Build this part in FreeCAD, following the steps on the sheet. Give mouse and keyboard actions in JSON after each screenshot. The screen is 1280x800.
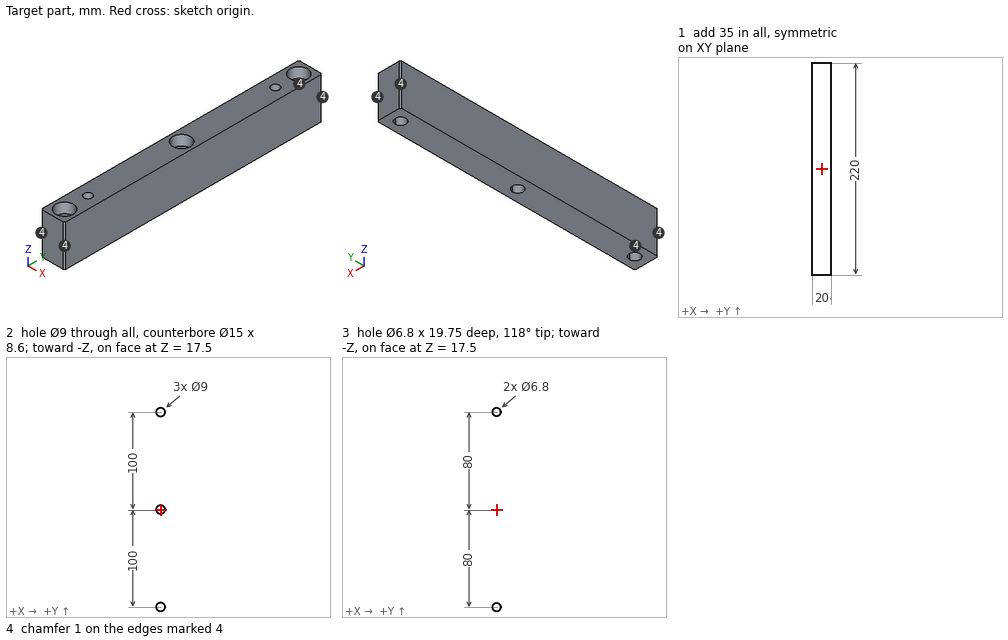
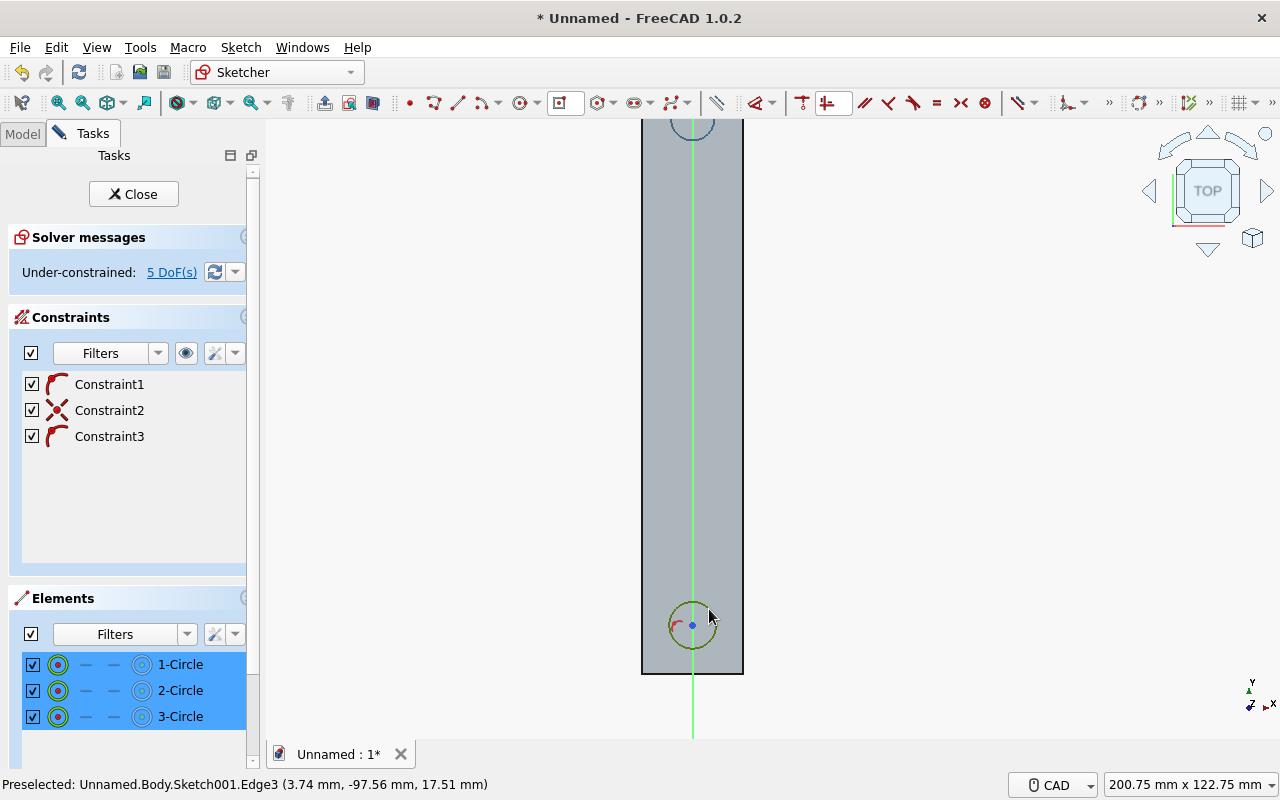
{"action": "key", "text": "e"}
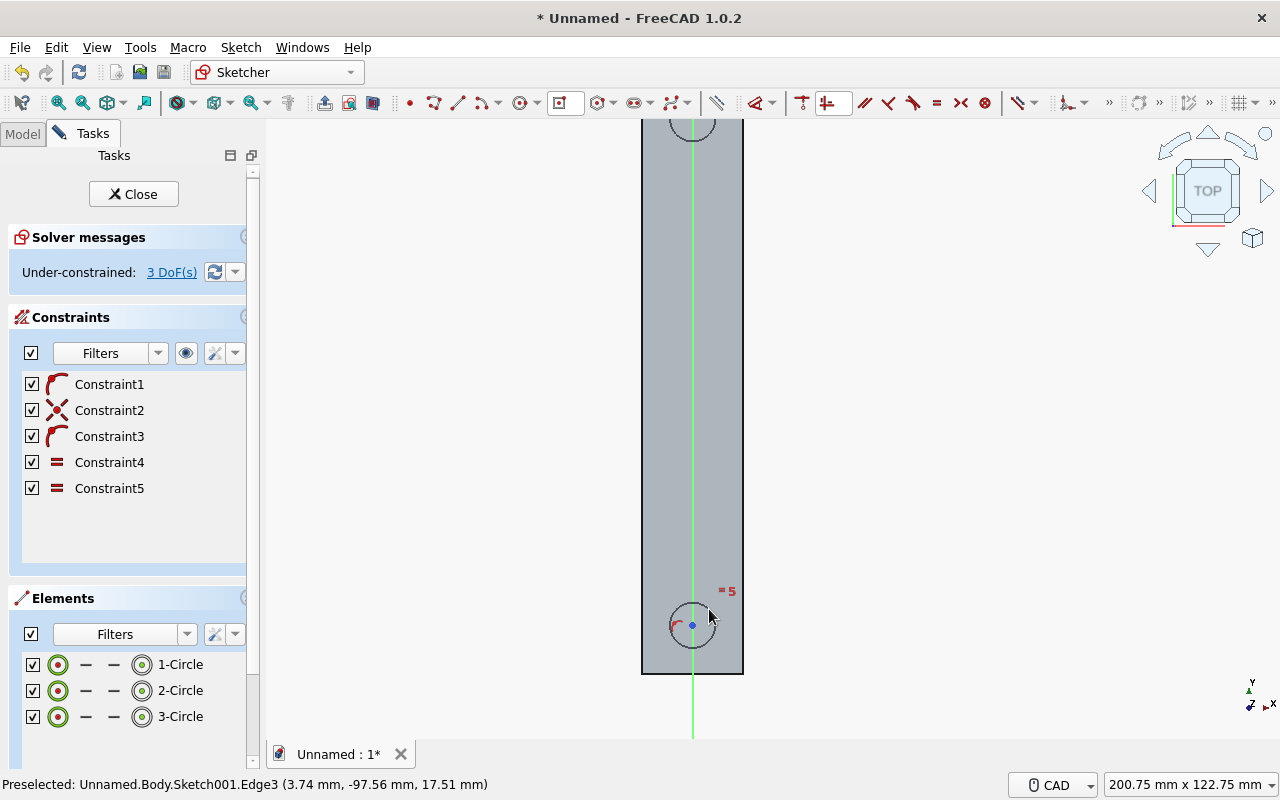
{"action": "left_click", "coordinate": [756, 104]}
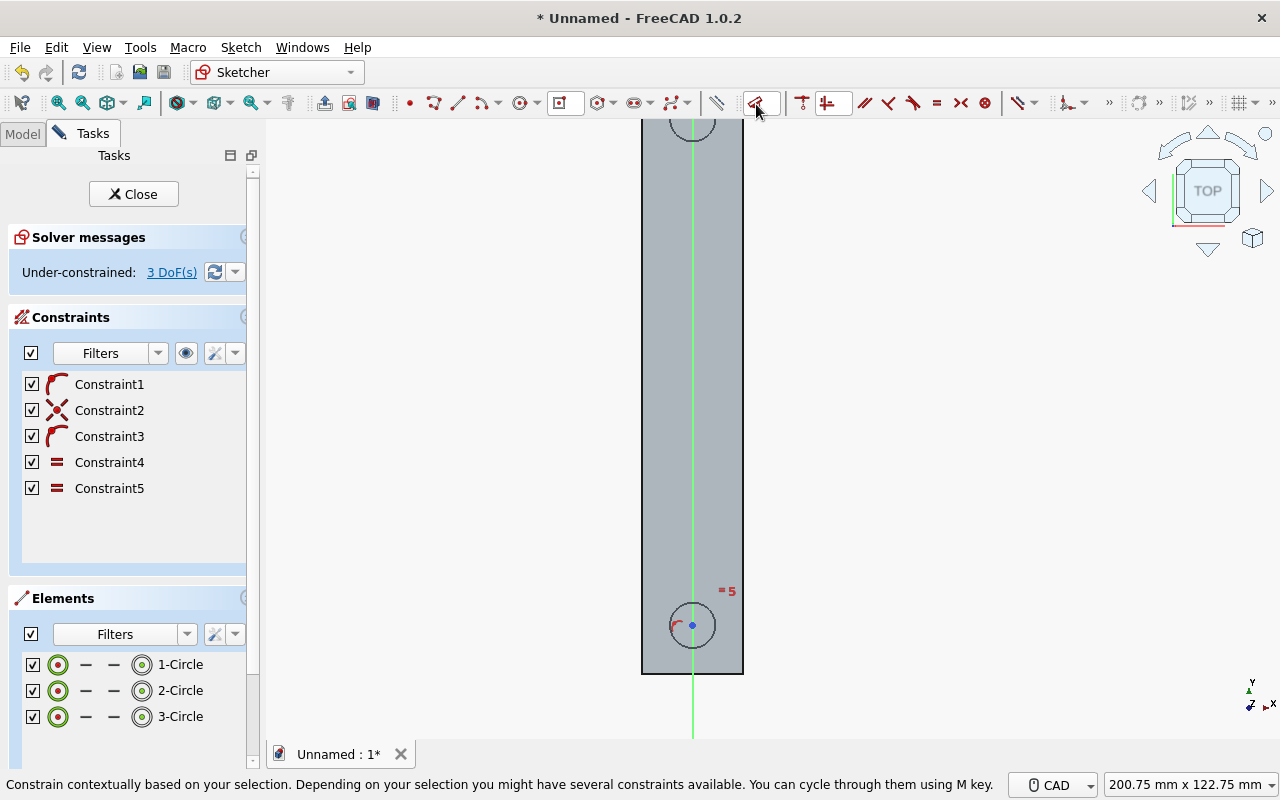
{"action": "scroll", "coordinate": [711, 610], "scroll_direction": "down", "scroll_amount": 5}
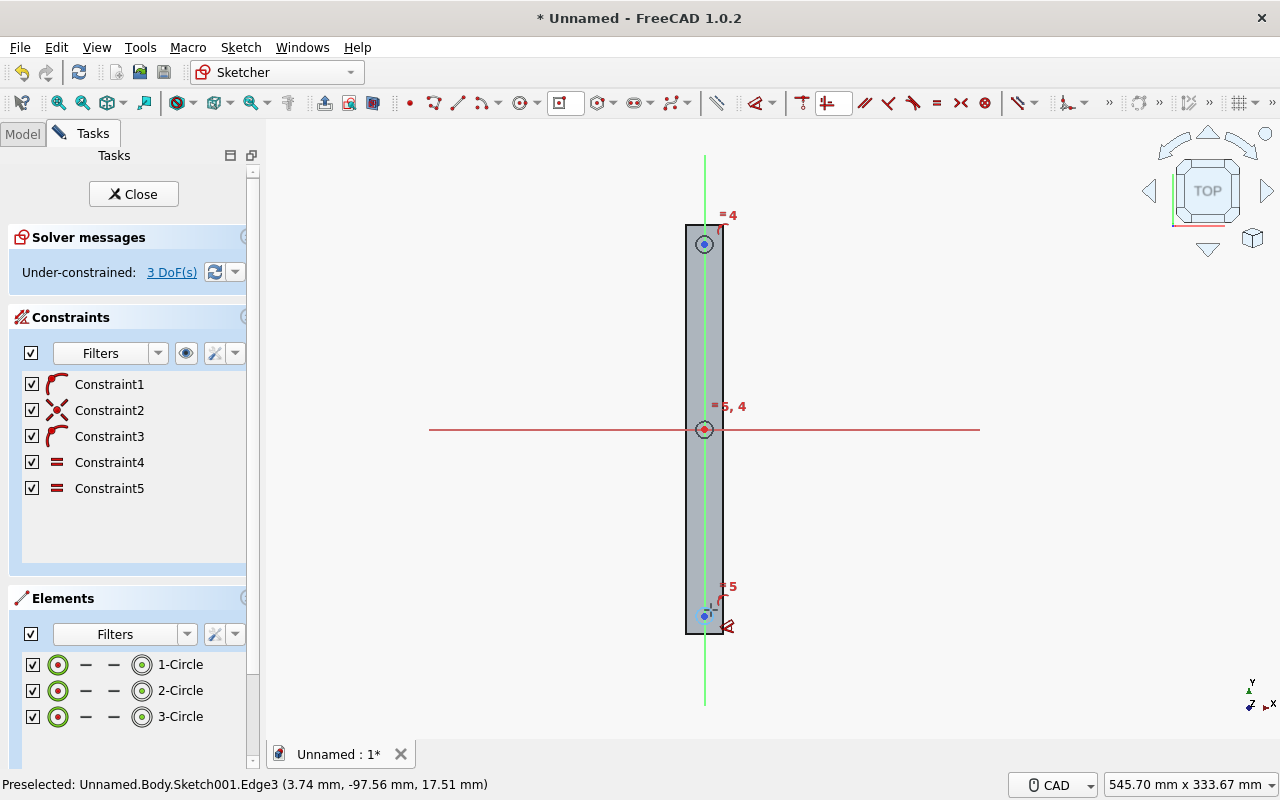
{"action": "scroll", "coordinate": [710, 239], "scroll_direction": "up", "scroll_amount": 5}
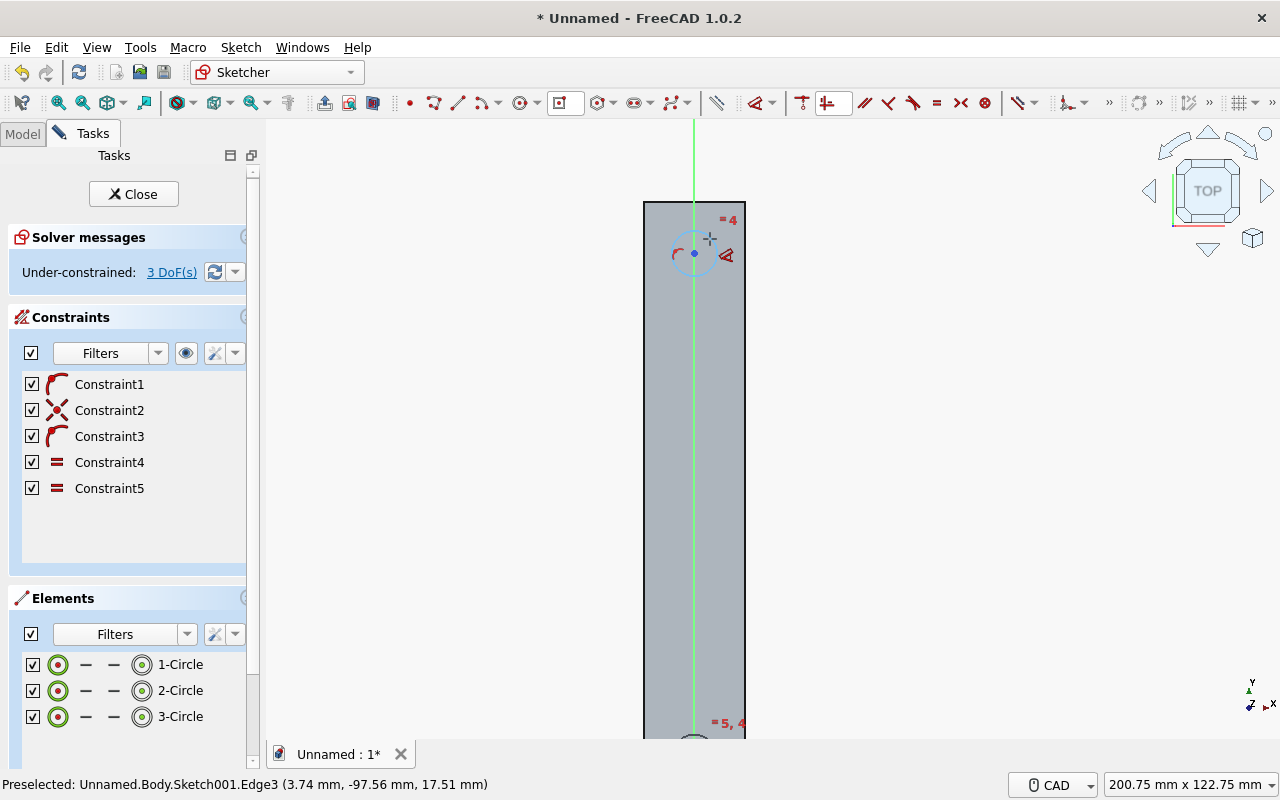
{"action": "left_click", "coordinate": [710, 238]}
{"action": "left_click", "coordinate": [733, 215]}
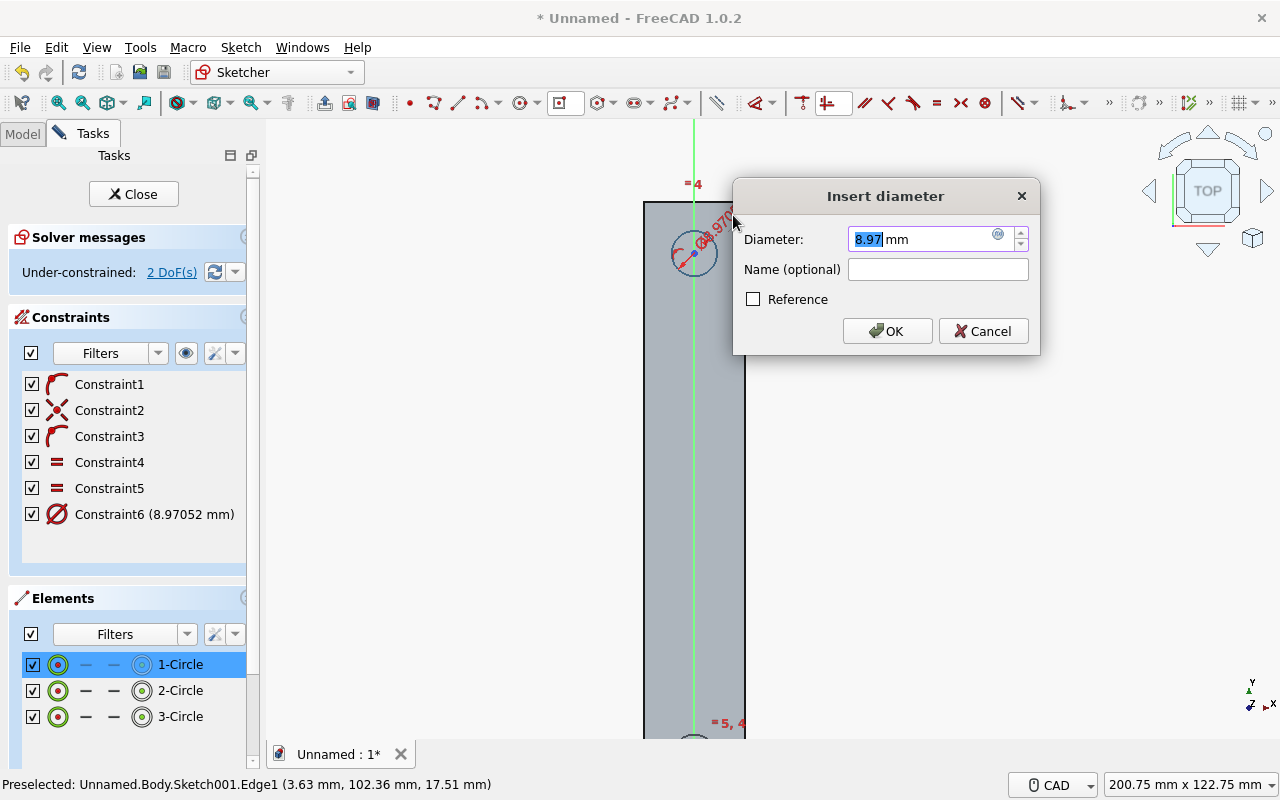
{"action": "type", "text": "9"}
{"action": "key", "text": "Return"}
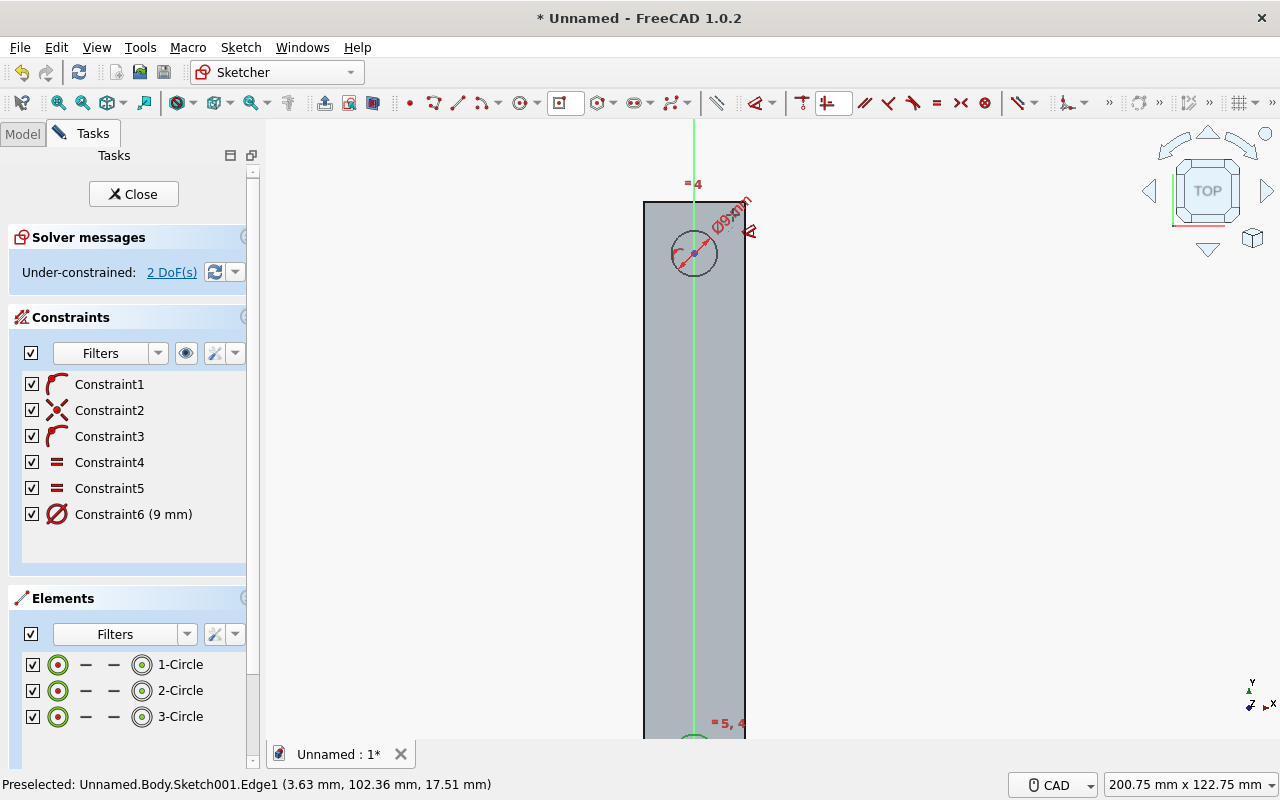
{"action": "left_click", "coordinate": [694, 254]}
{"action": "left_click", "coordinate": [728, 482]}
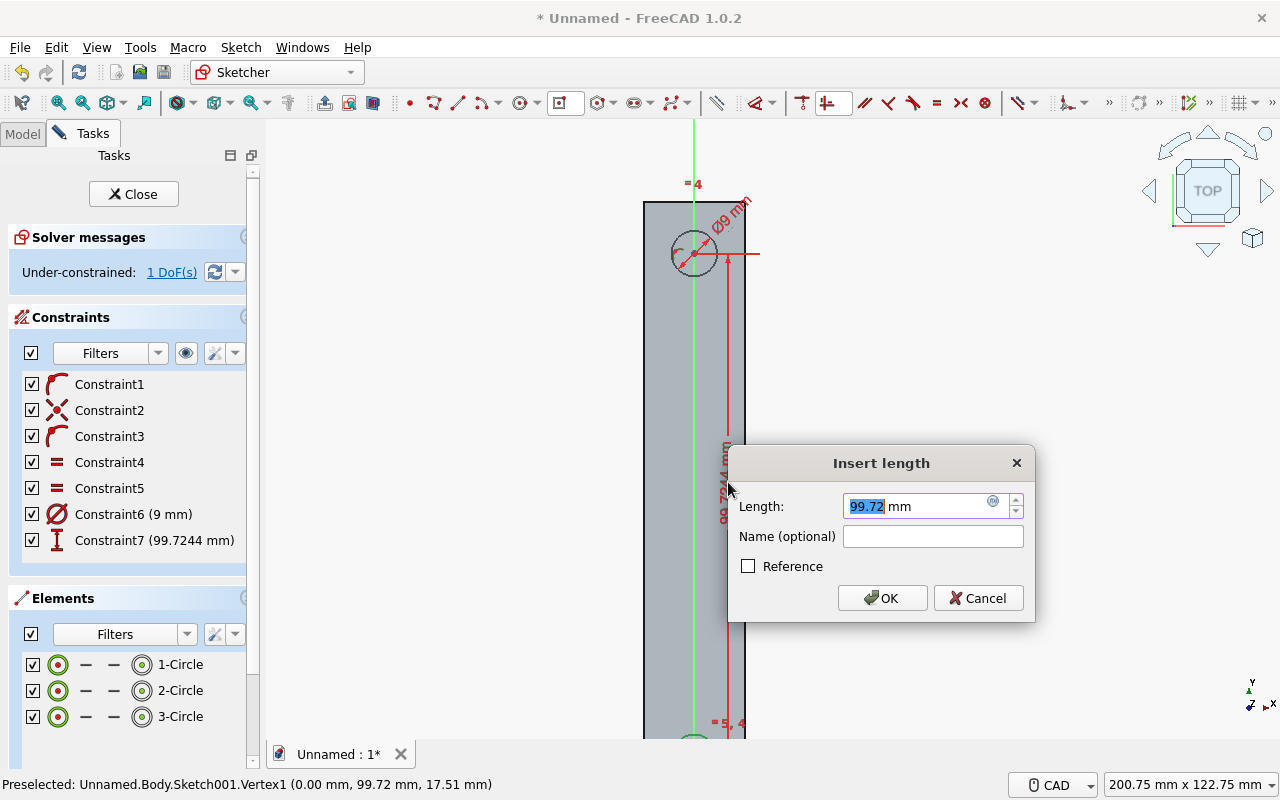
{"action": "type", "text": "100"}
{"action": "key", "text": "Return"}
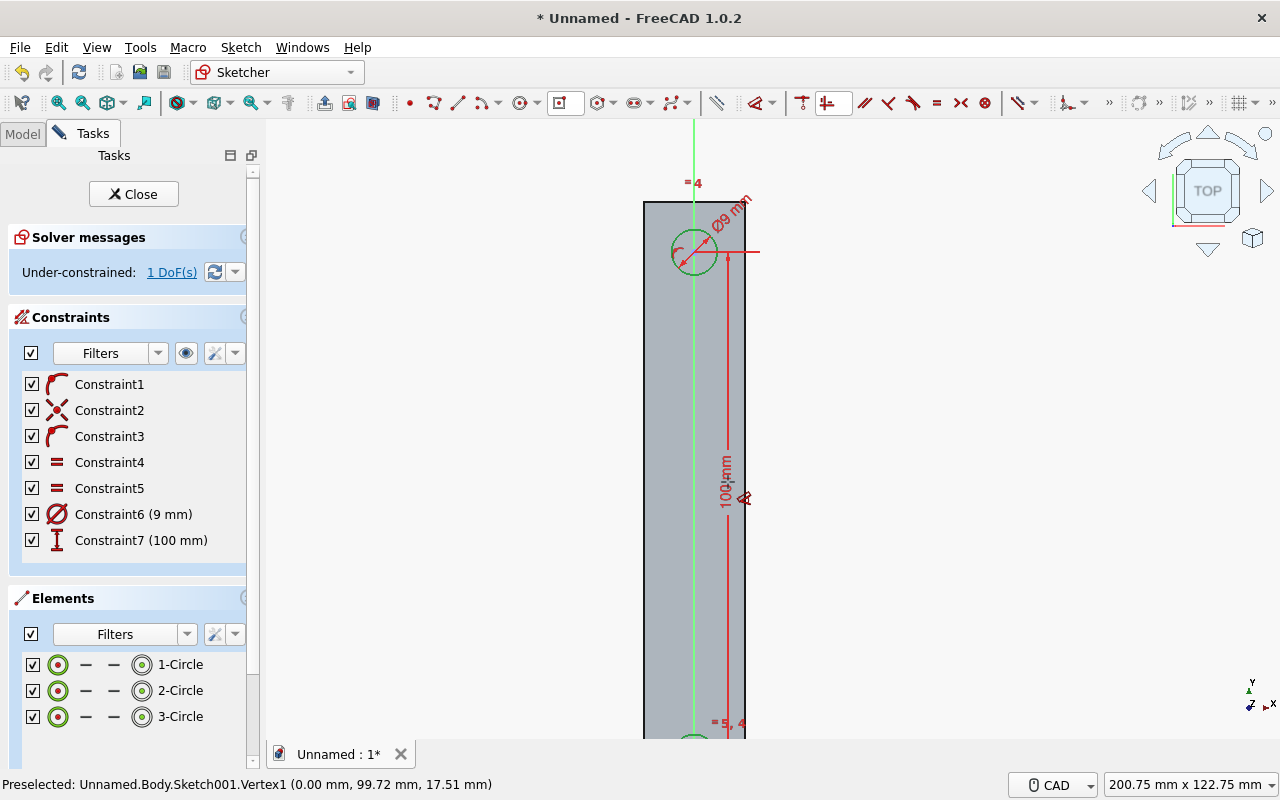
{"action": "scroll", "coordinate": [710, 238], "scroll_direction": "down", "scroll_amount": 5}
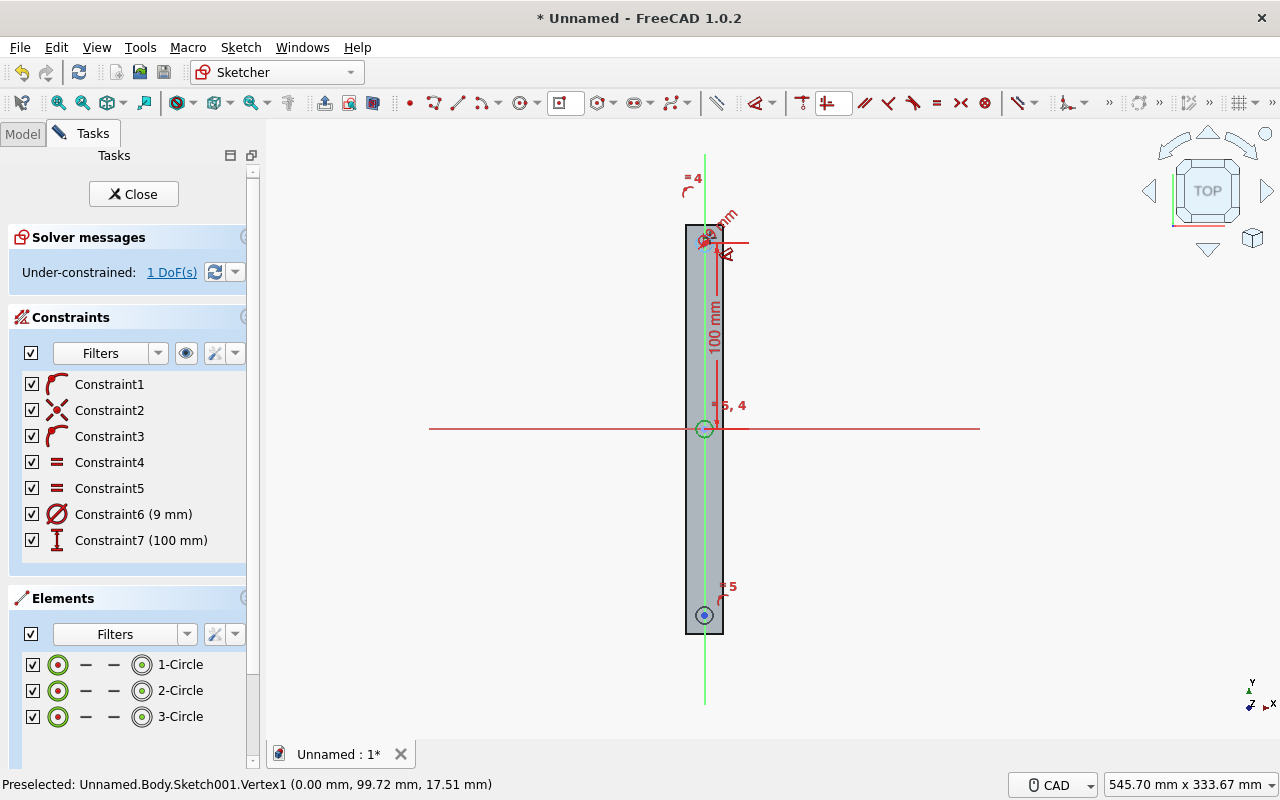
{"action": "left_click", "coordinate": [705, 616]}
{"action": "left_click", "coordinate": [739, 522]}